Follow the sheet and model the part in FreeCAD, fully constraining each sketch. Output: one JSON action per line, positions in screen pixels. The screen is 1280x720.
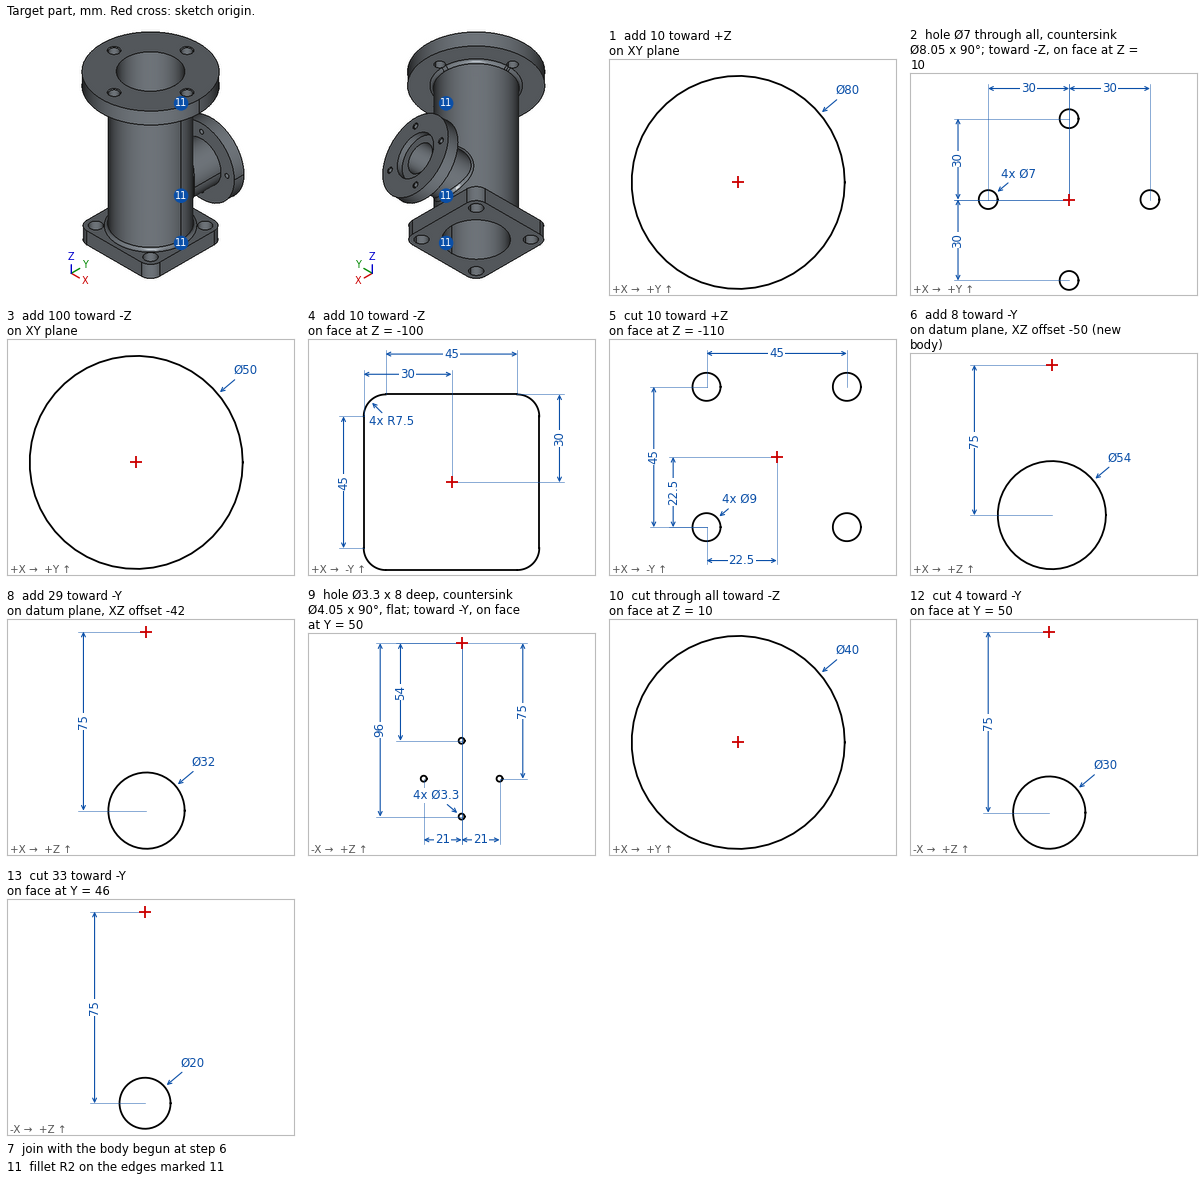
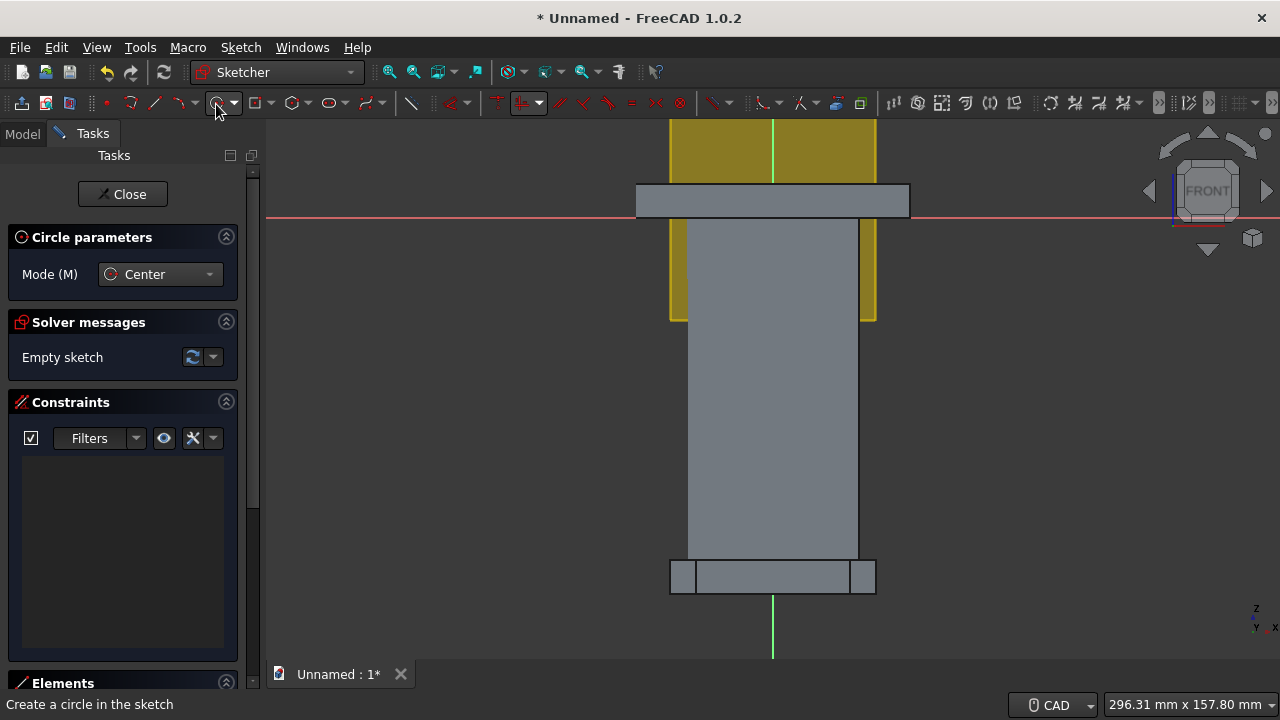
{"action": "left_click", "coordinate": [773, 475]}
{"action": "mouse_move", "coordinate": [838, 409]}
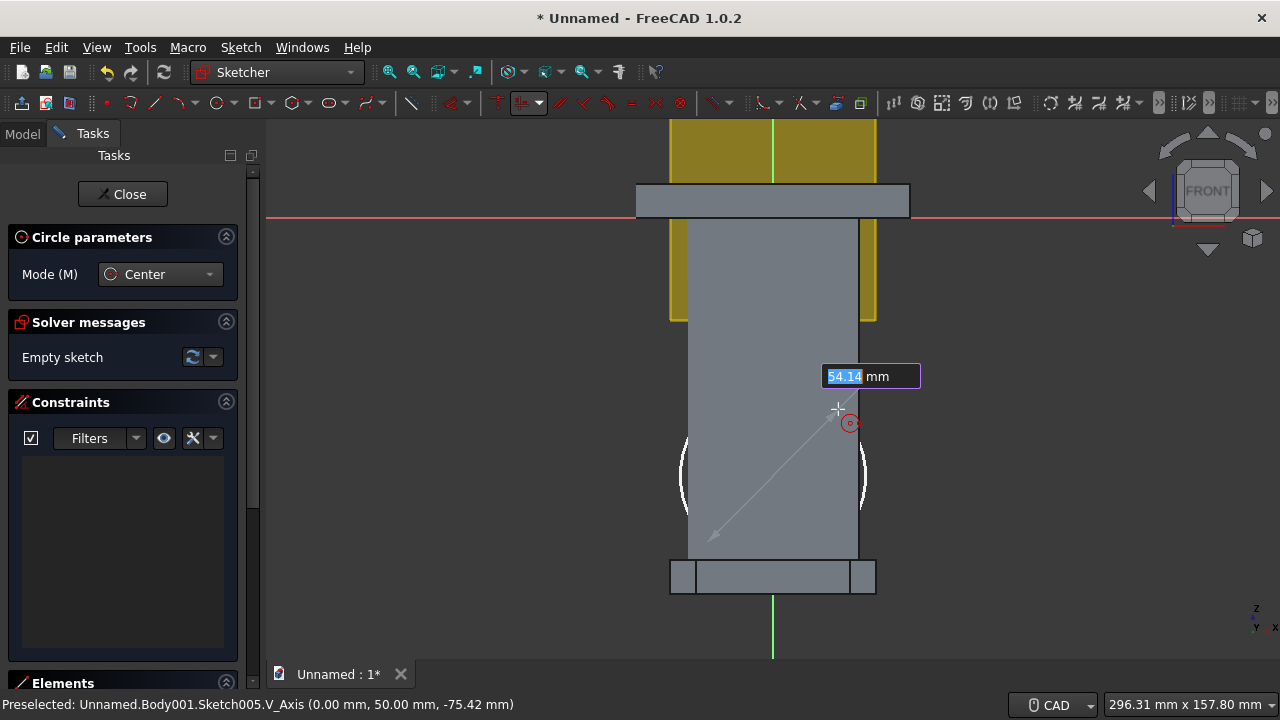
{"action": "type", "text": "54"}
{"action": "key", "text": "Return"}
{"action": "key", "text": "Escape"}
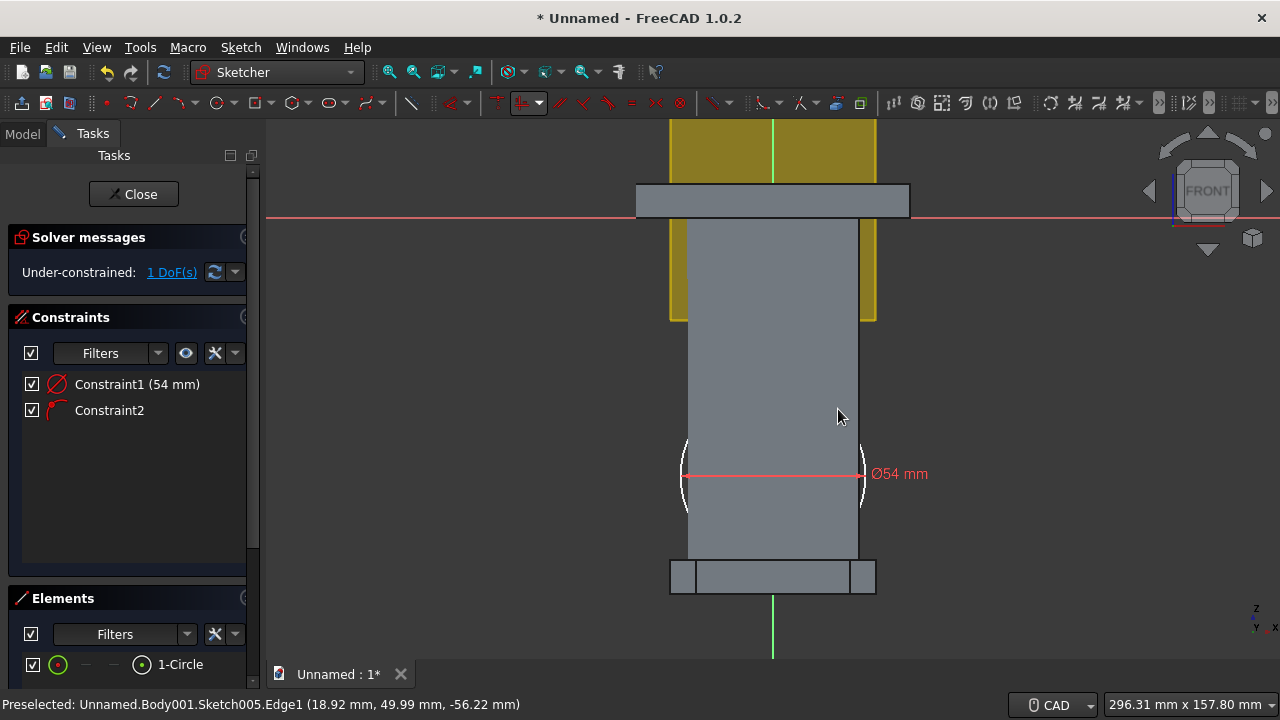
{"action": "left_click", "coordinate": [450, 104]}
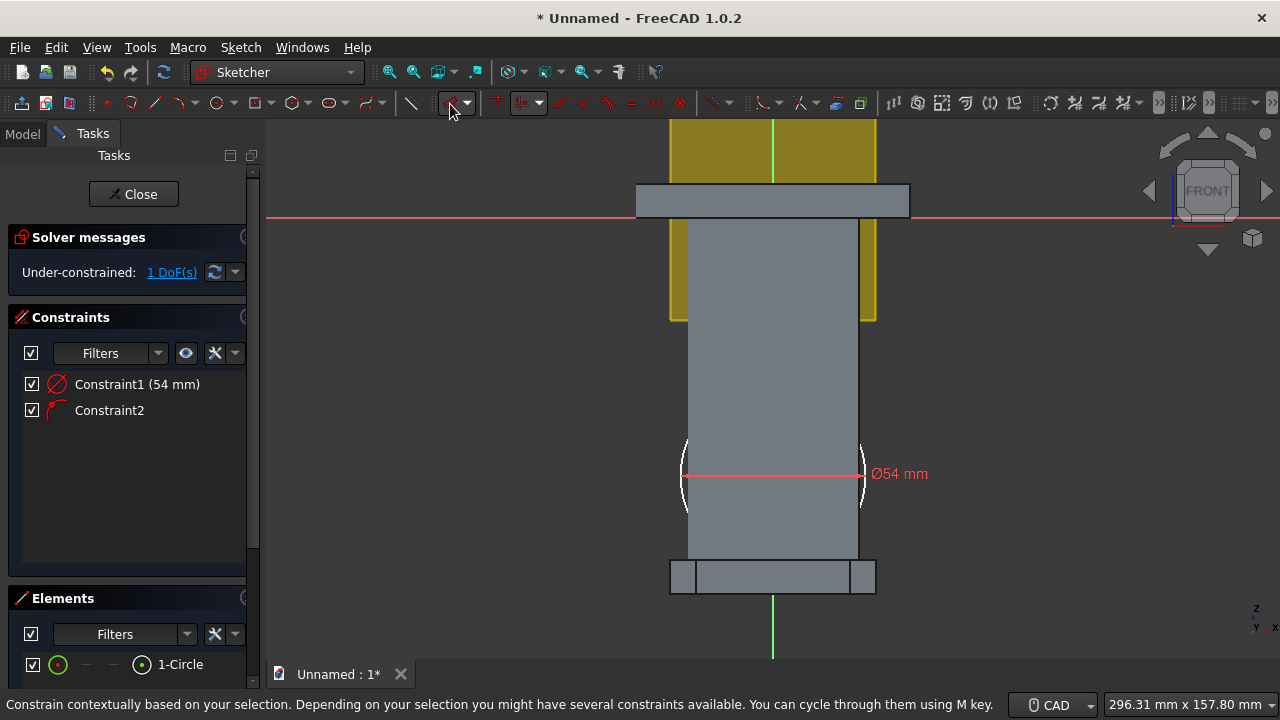
{"action": "left_click", "coordinate": [773, 476]}
{"action": "left_click", "coordinate": [807, 347]}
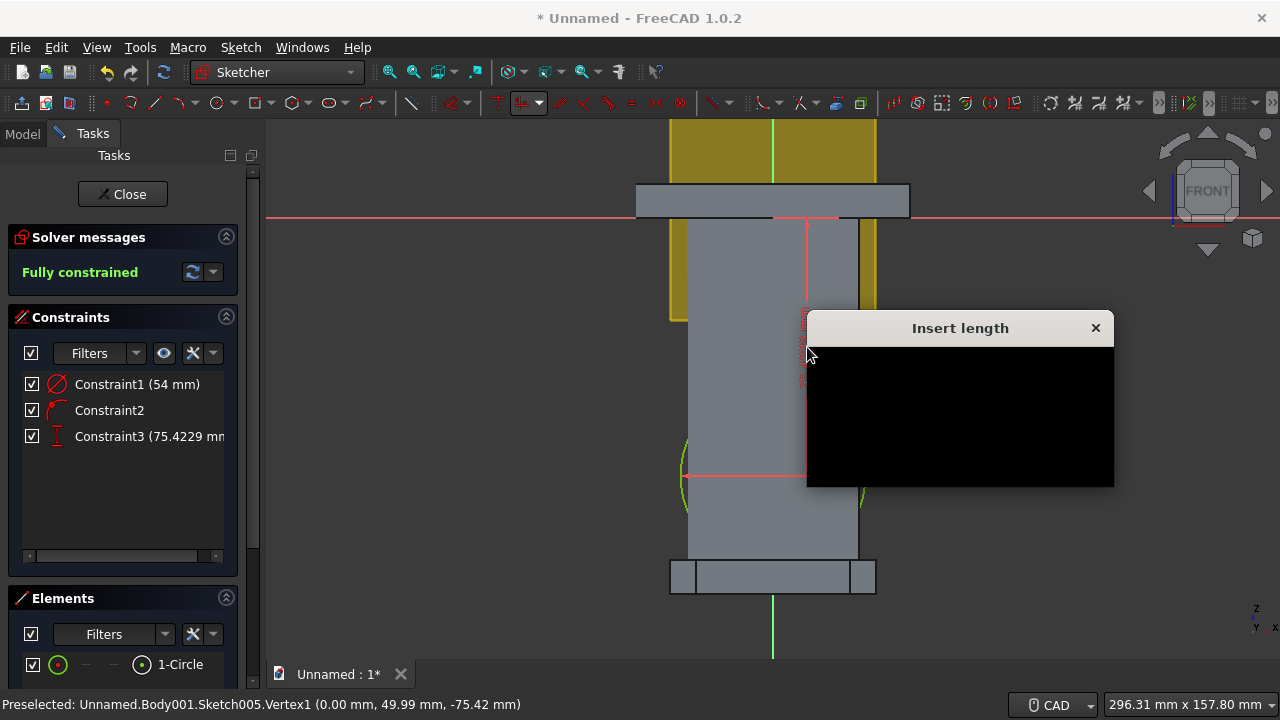
{"action": "type", "text": "75"}
{"action": "key", "text": "Return"}
{"action": "key", "text": "Escape"}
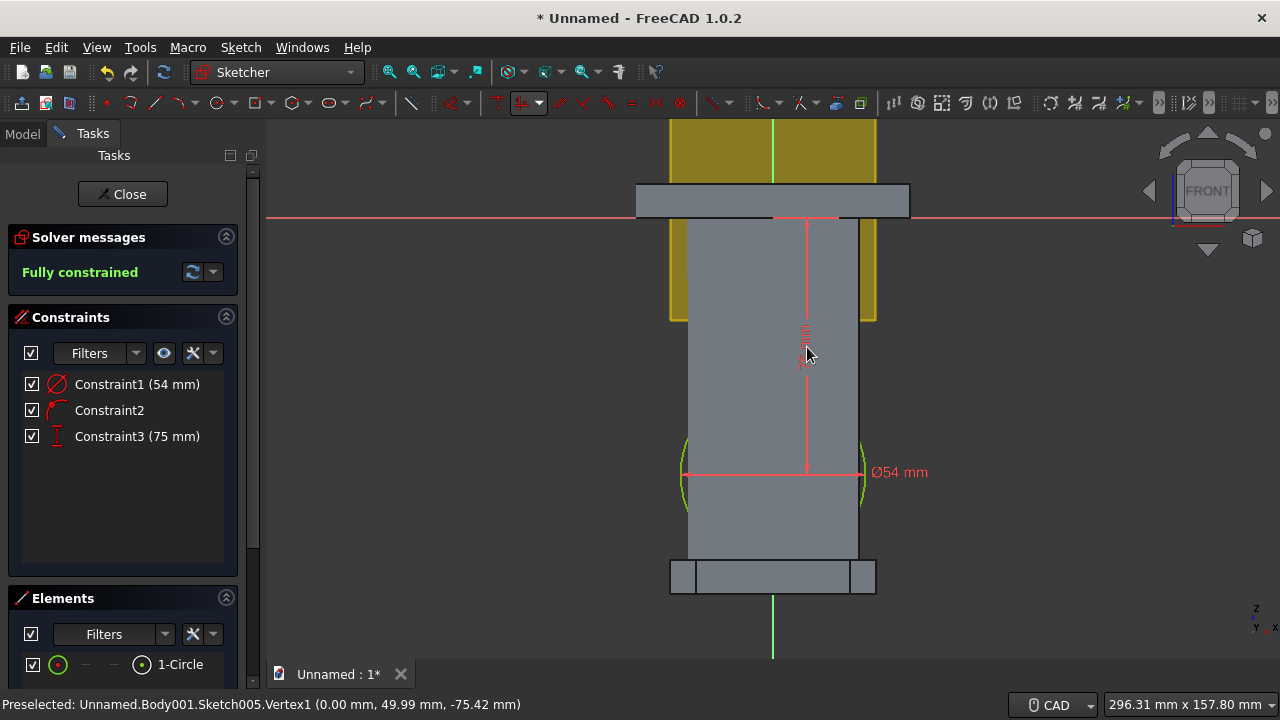
{"action": "left_click", "coordinate": [123, 194]}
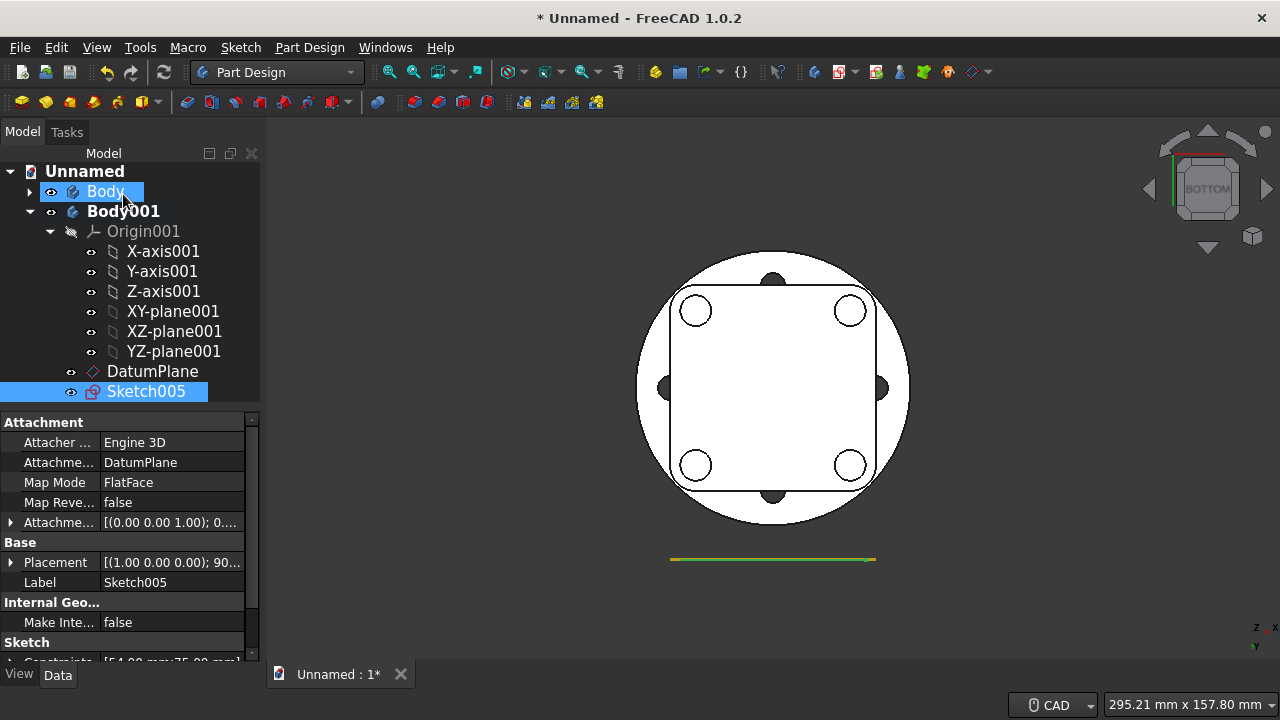
{"action": "left_click", "coordinate": [22, 102]}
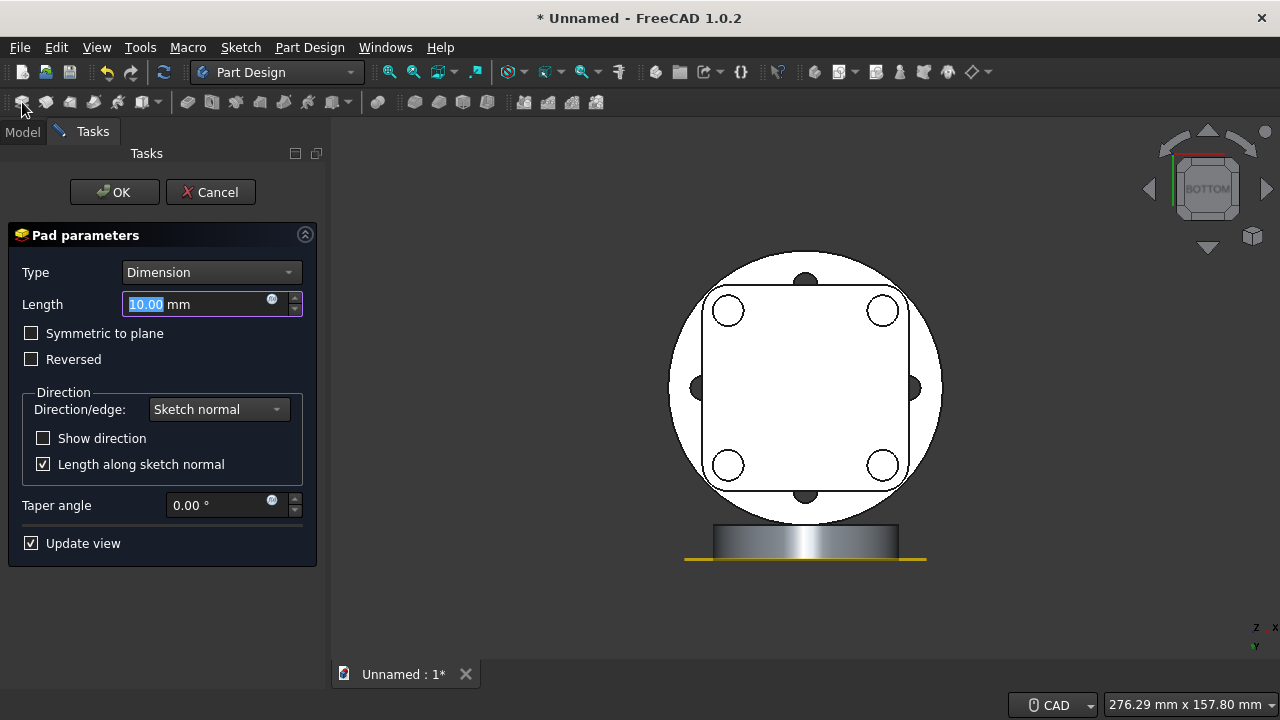
{"action": "type", "text": "8"}
{"action": "key", "text": "Tab"}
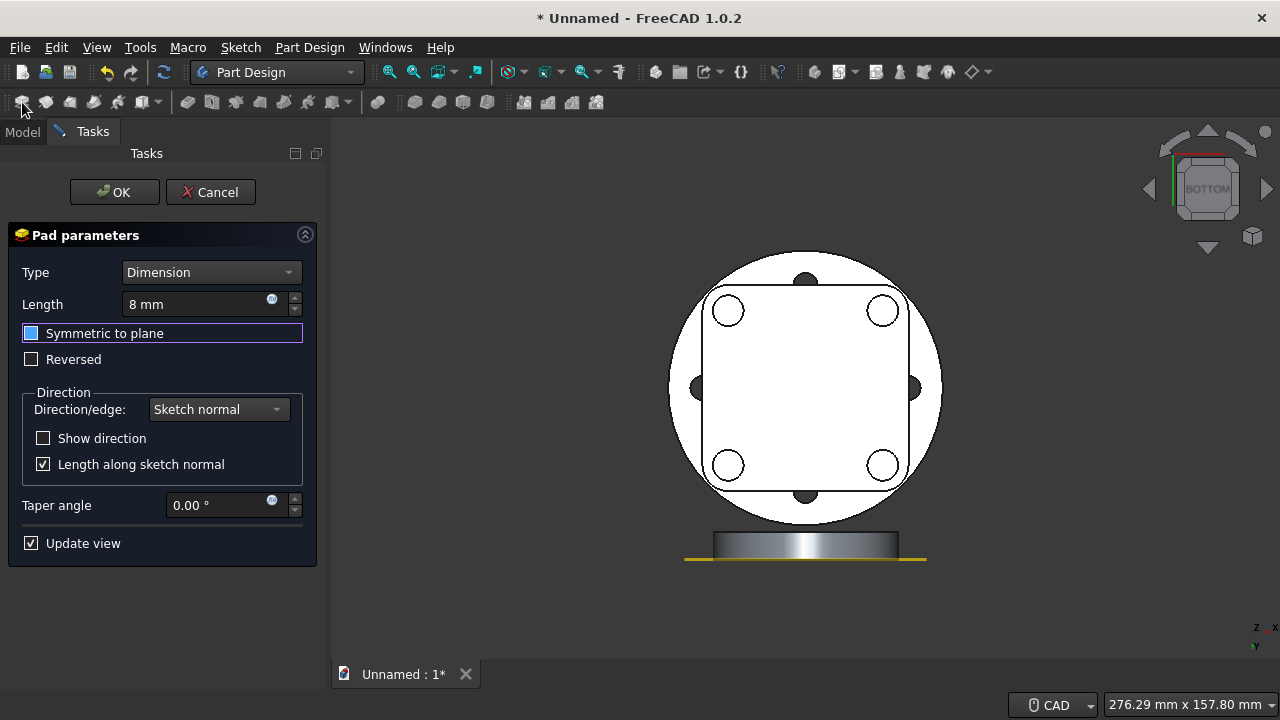
{"action": "left_click", "coordinate": [115, 192]}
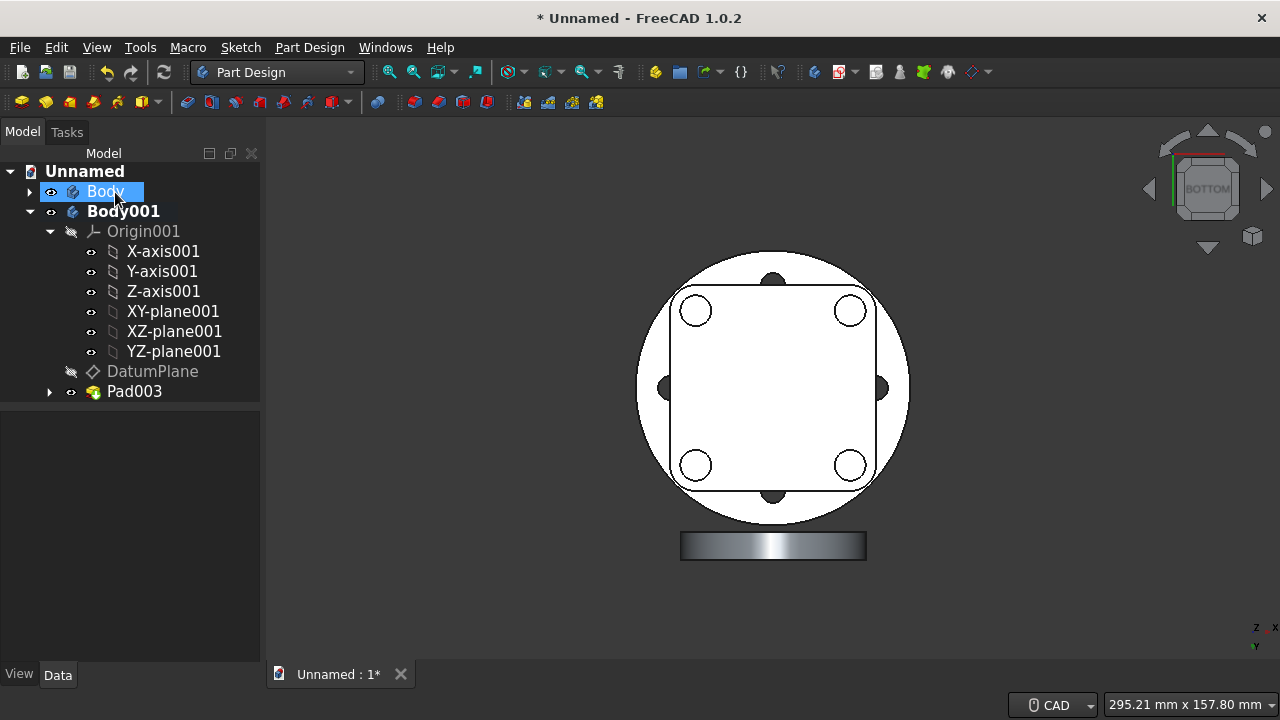
{"action": "left_click", "coordinate": [390, 72]}